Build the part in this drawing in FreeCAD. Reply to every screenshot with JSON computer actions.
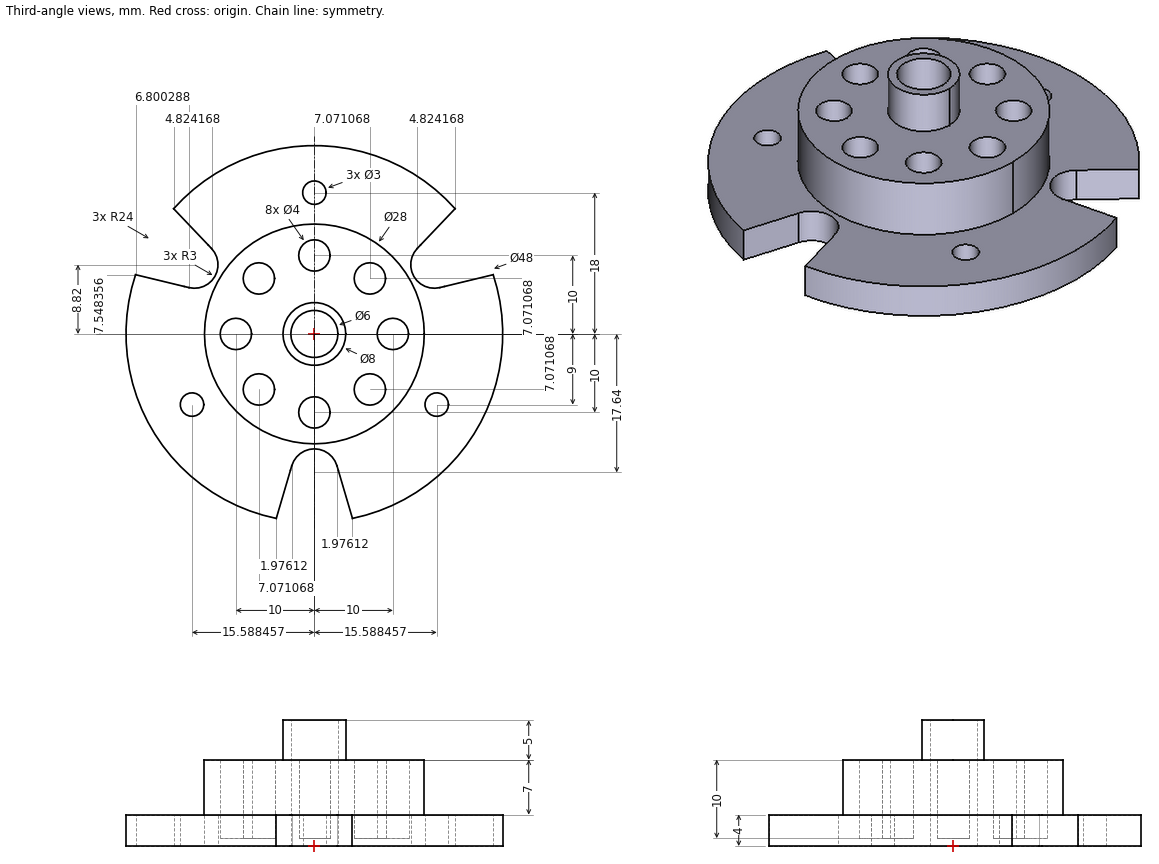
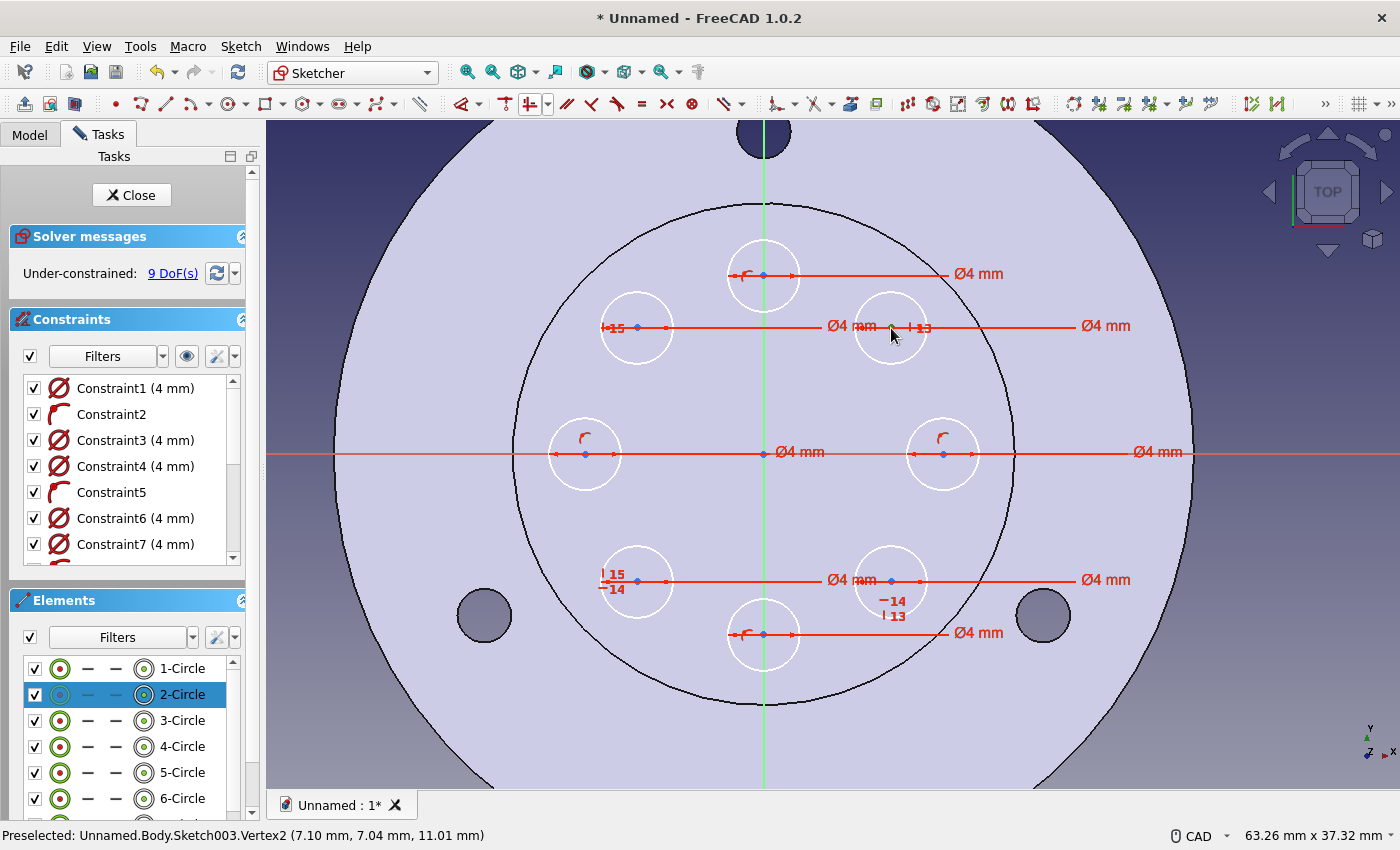
{"action": "left_click", "coordinate": [637, 328]}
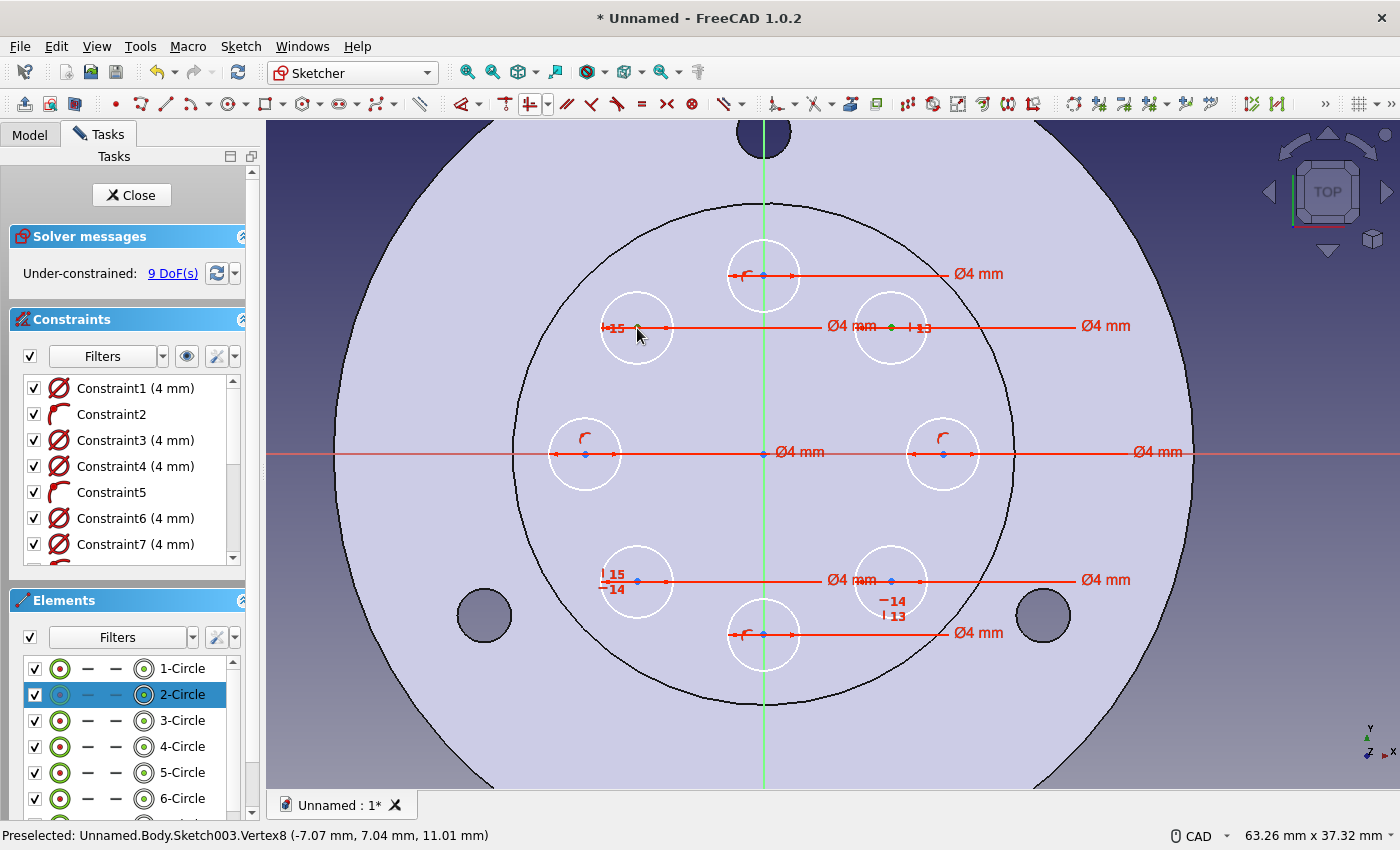
{"action": "left_click", "coordinate": [548, 104]}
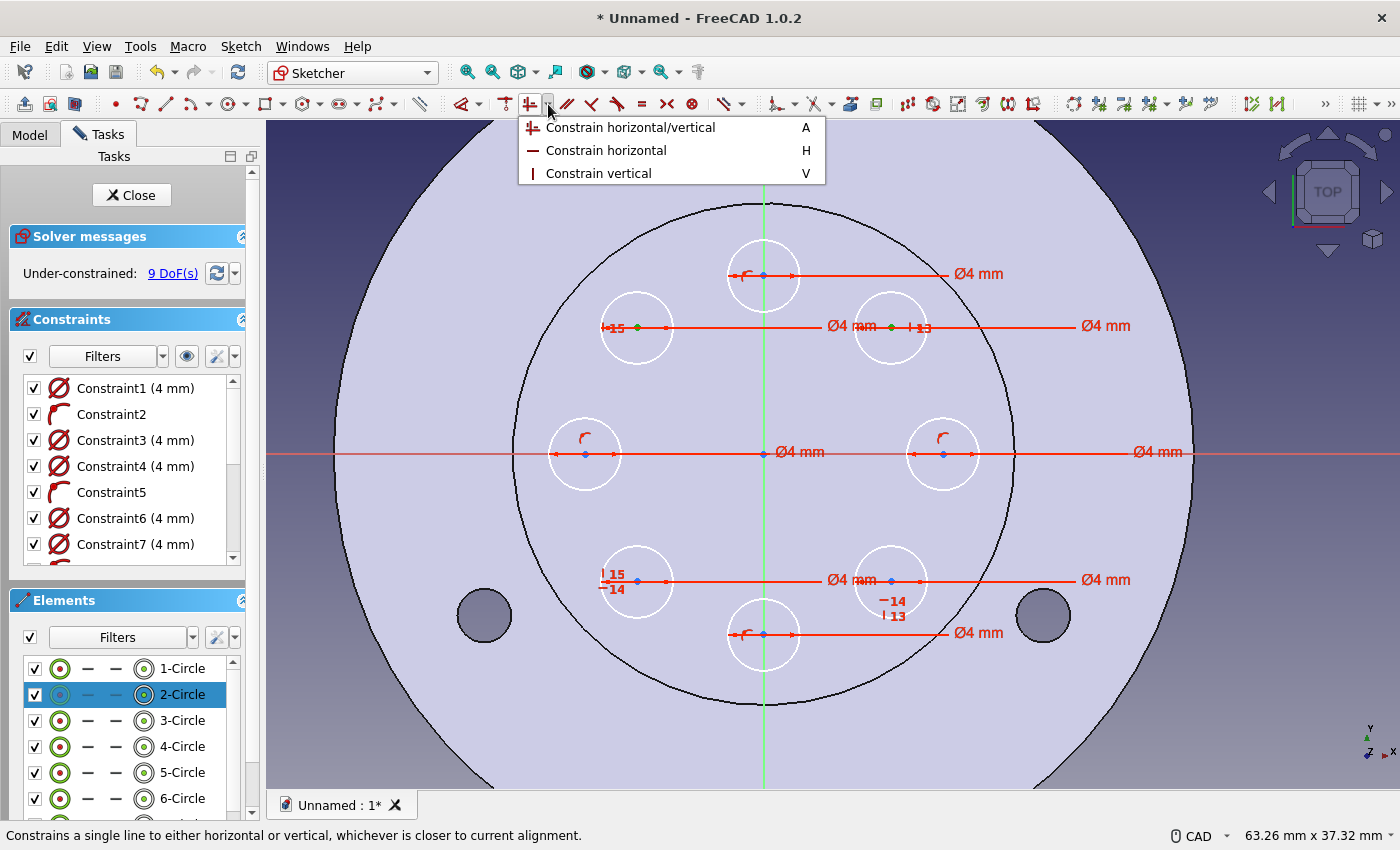
{"action": "left_click", "coordinate": [672, 150]}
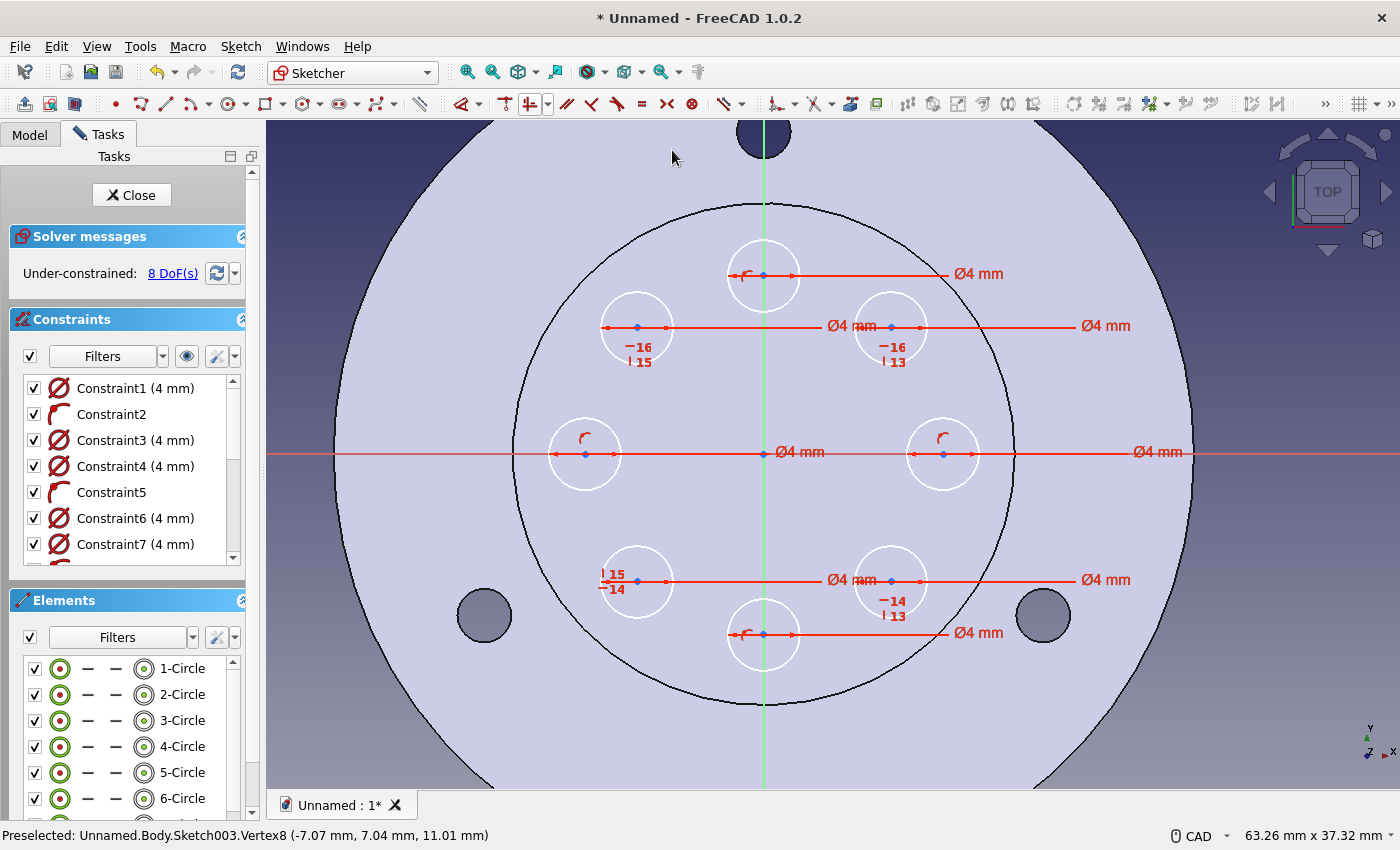
{"action": "key", "text": "d"}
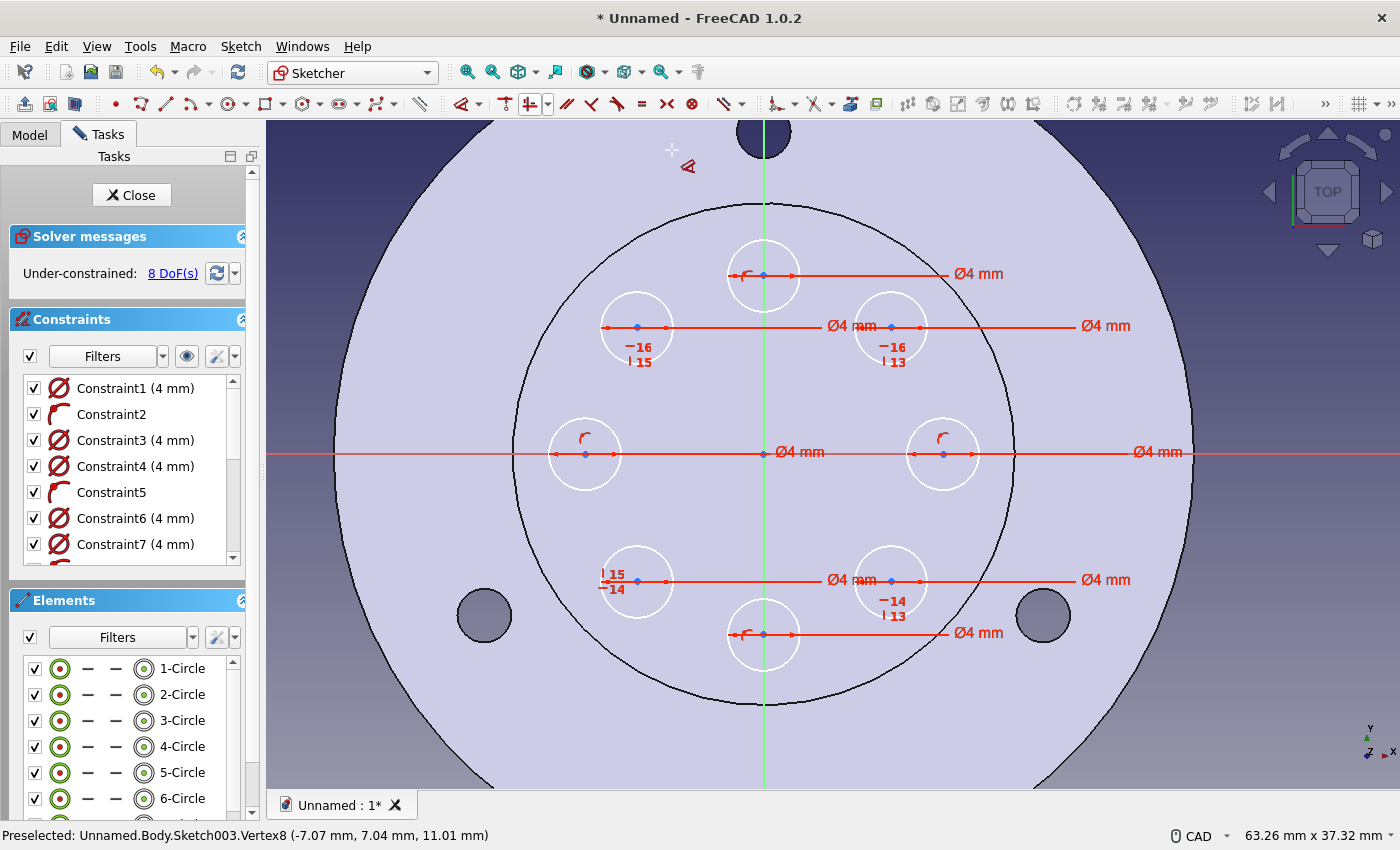
{"action": "left_click", "coordinate": [764, 276]}
{"action": "left_click", "coordinate": [798, 365]}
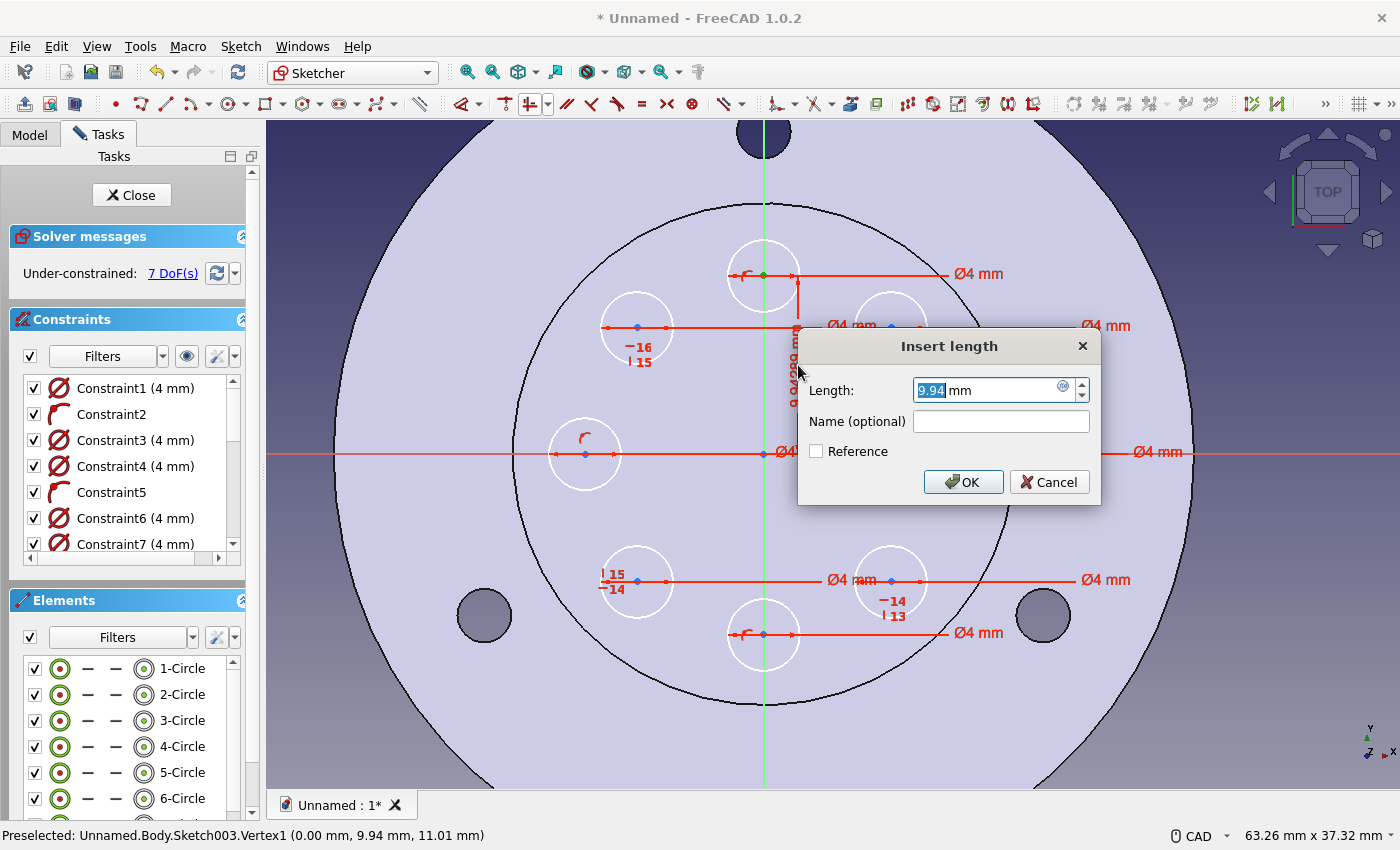
{"action": "type", "text": "10"}
{"action": "key", "text": "Return"}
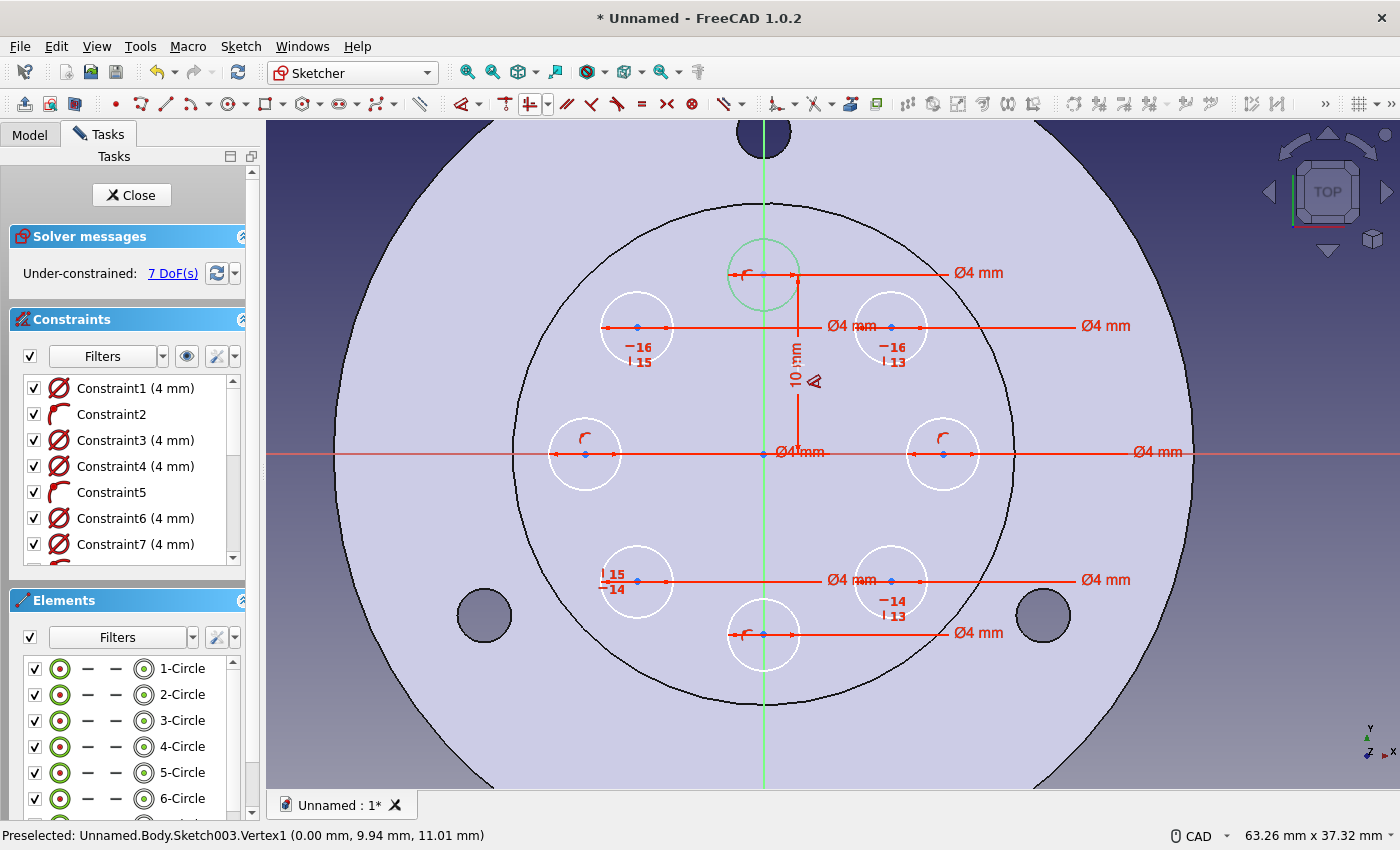
{"action": "left_click", "coordinate": [943, 454]}
{"action": "left_click", "coordinate": [853, 488]}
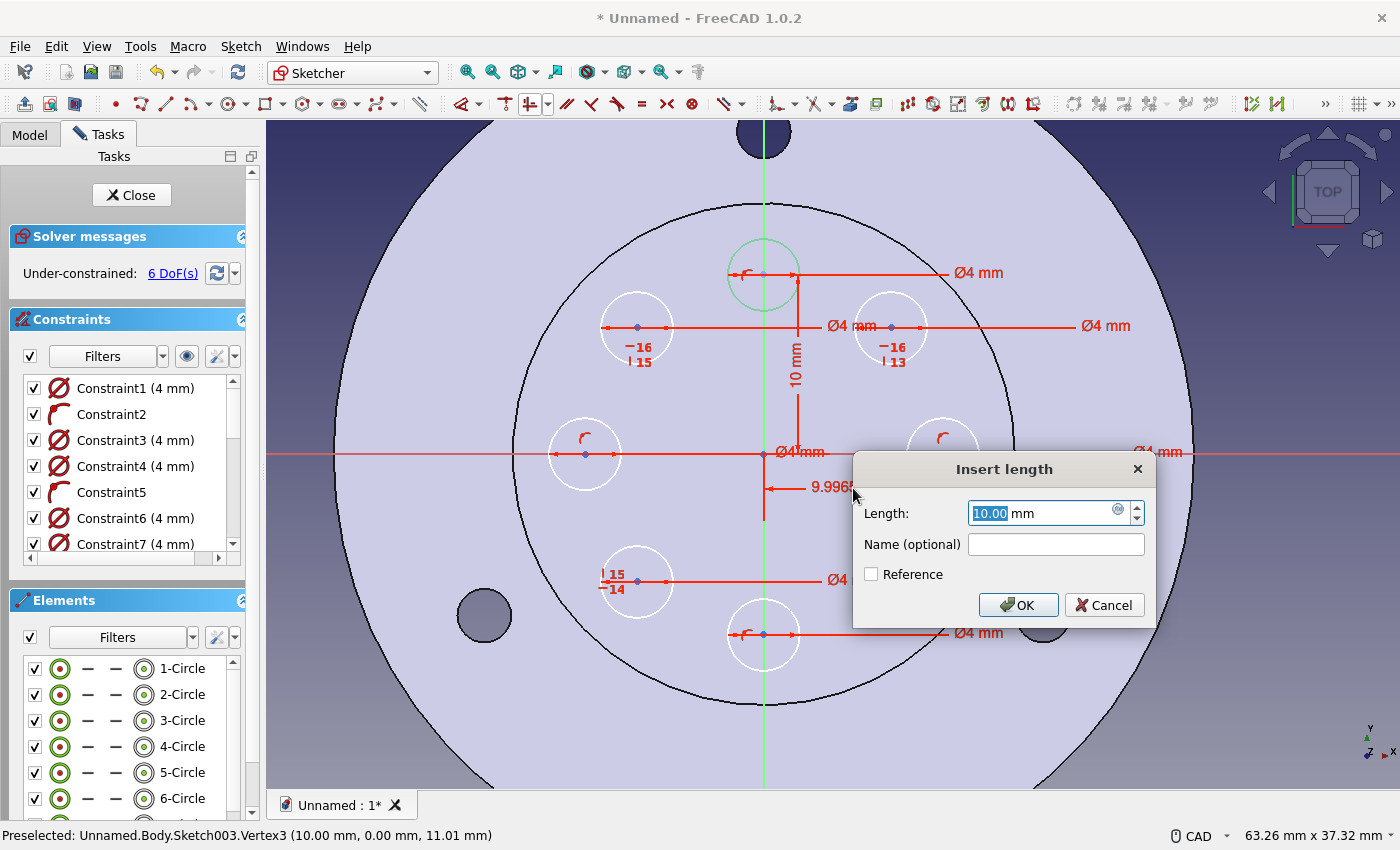
{"action": "type", "text": "10"}
{"action": "key", "text": "Return"}